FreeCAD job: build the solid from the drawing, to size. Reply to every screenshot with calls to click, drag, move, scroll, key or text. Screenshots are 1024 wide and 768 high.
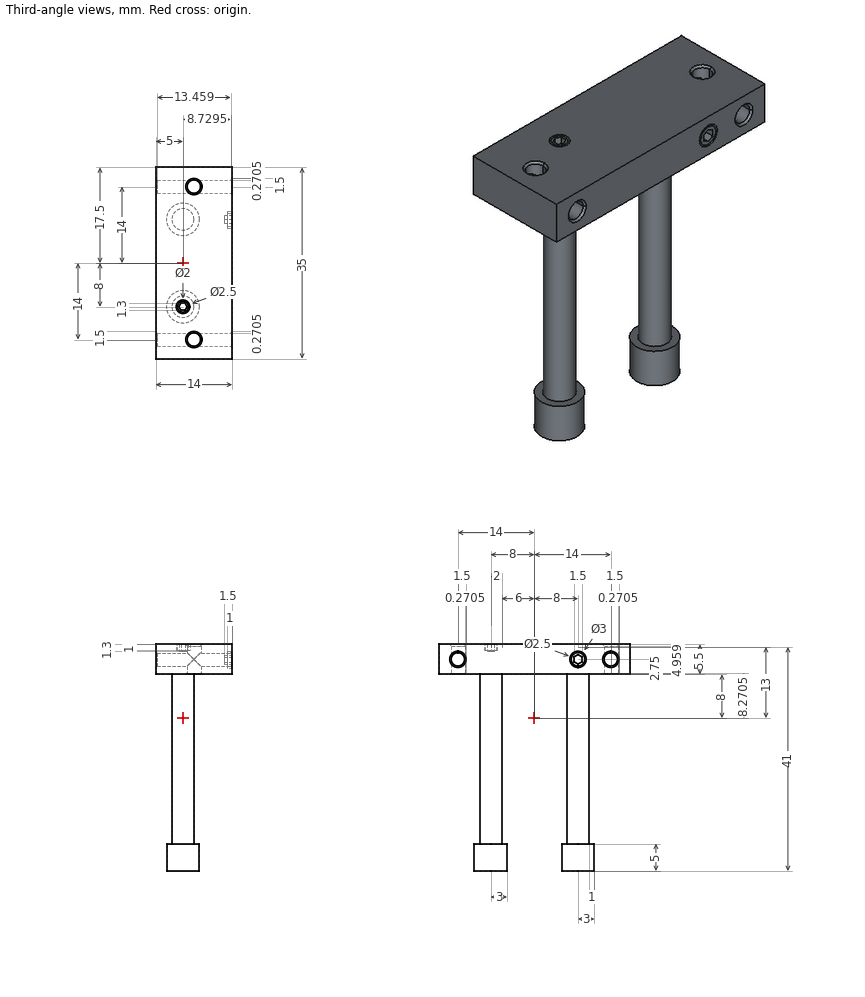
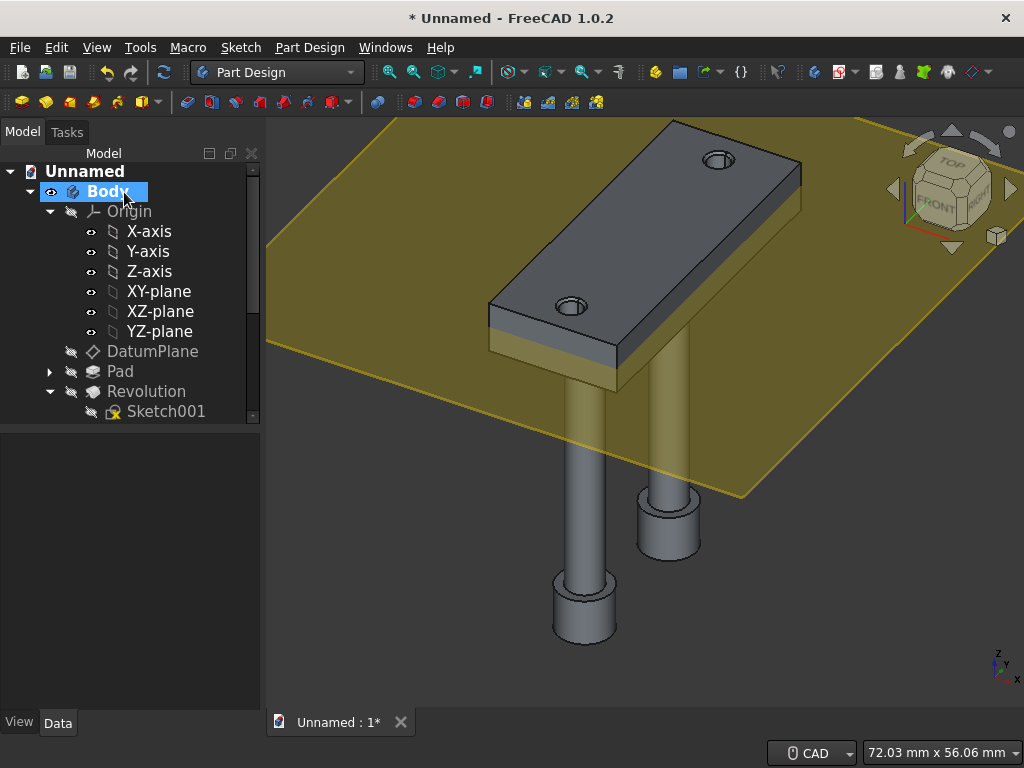
scroll(100, 287, down, 3)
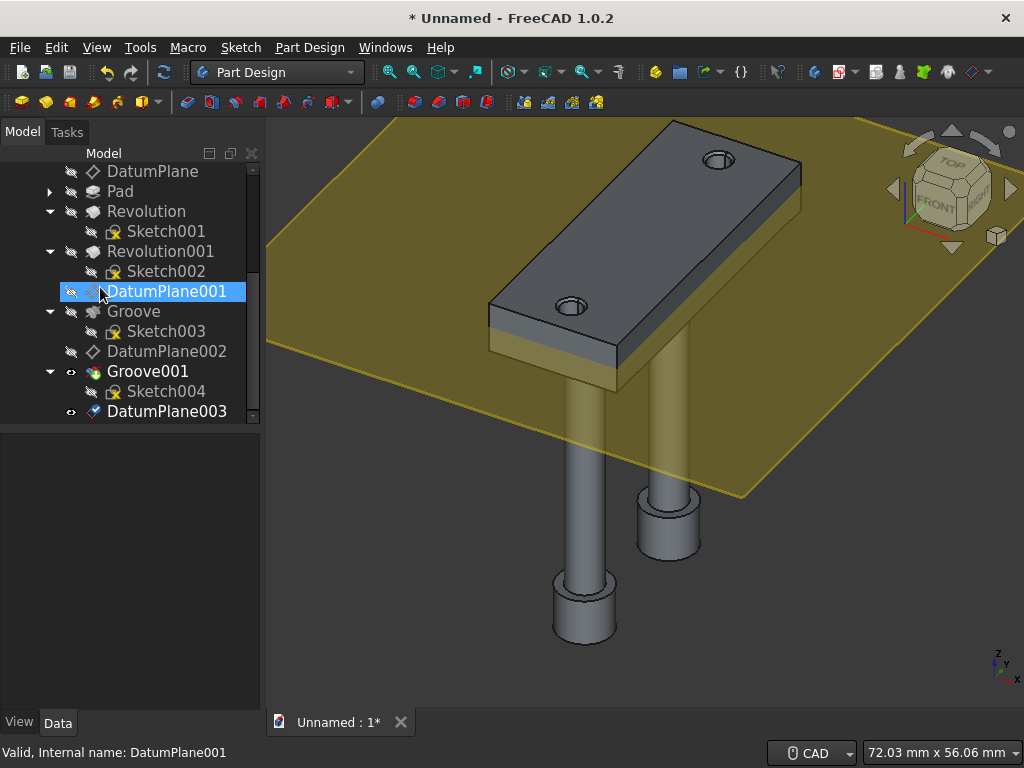
click(116, 412)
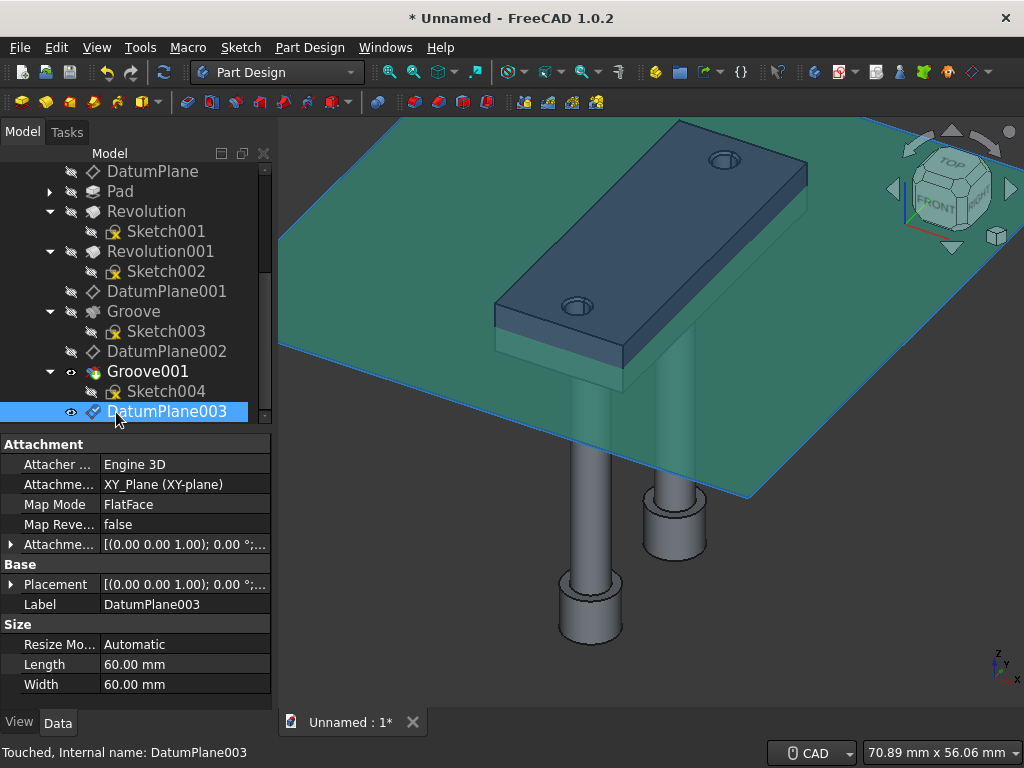
click(840, 72)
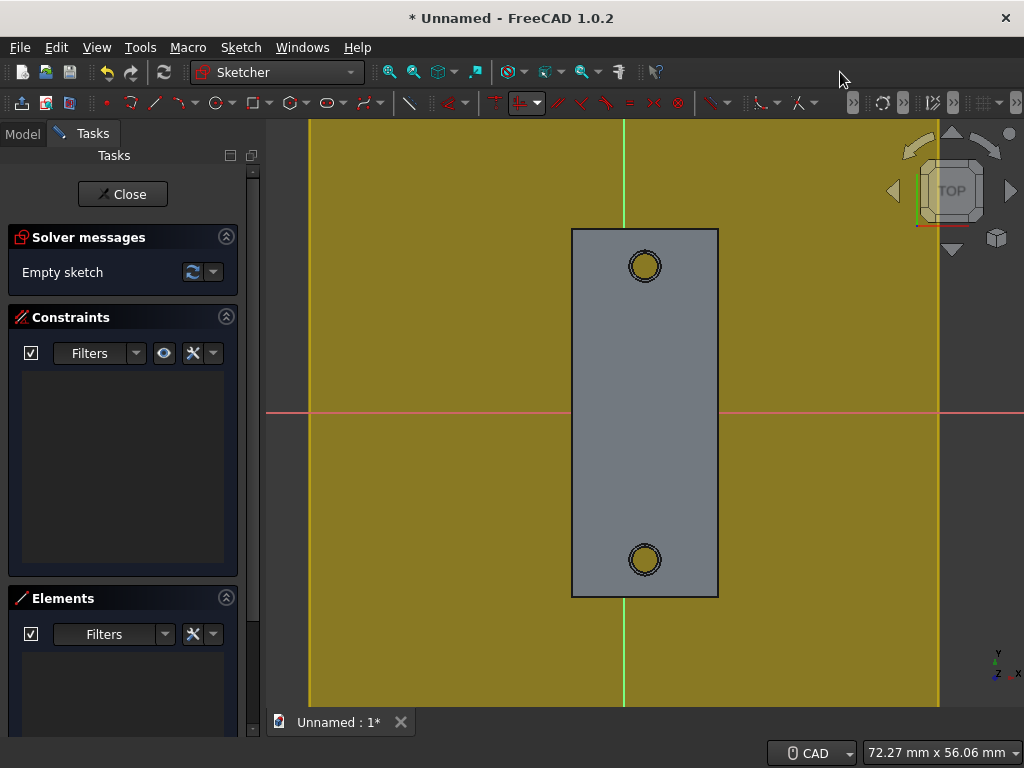
click(70, 104)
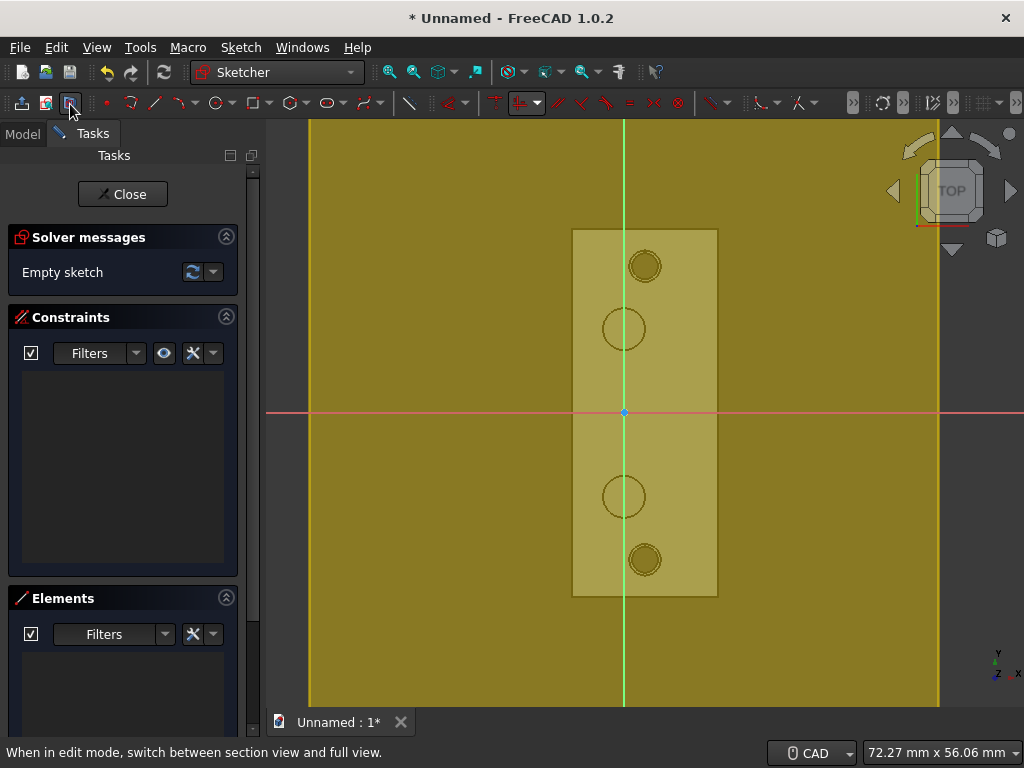
scroll(663, 233, up, 3)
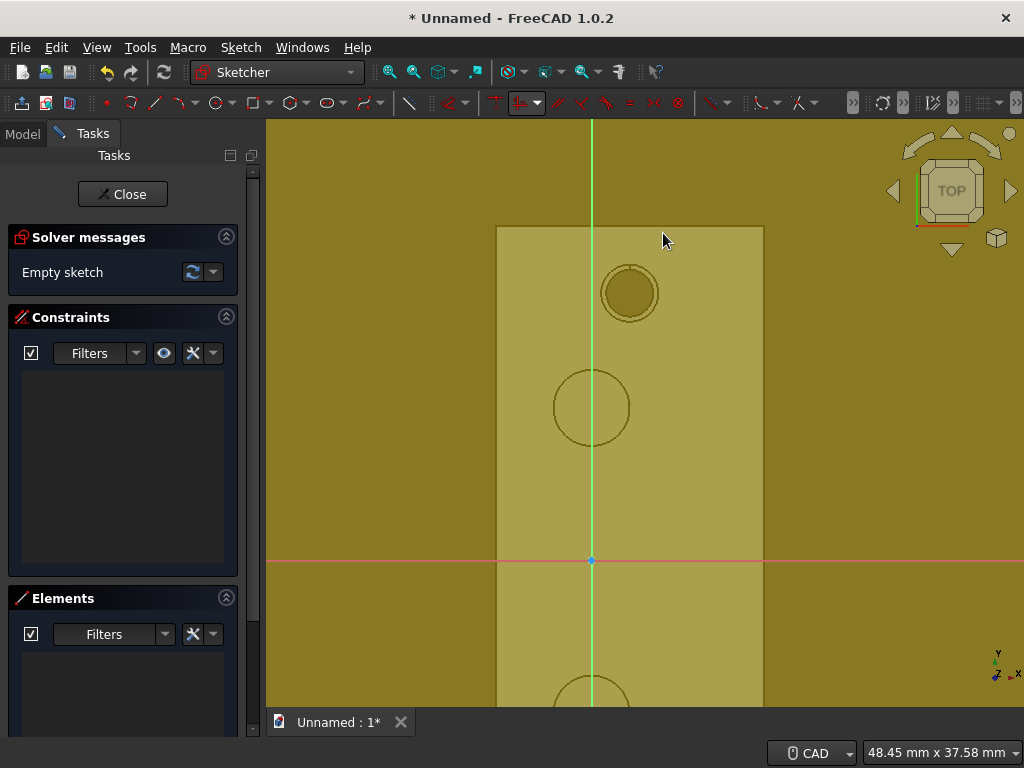
click(132, 104)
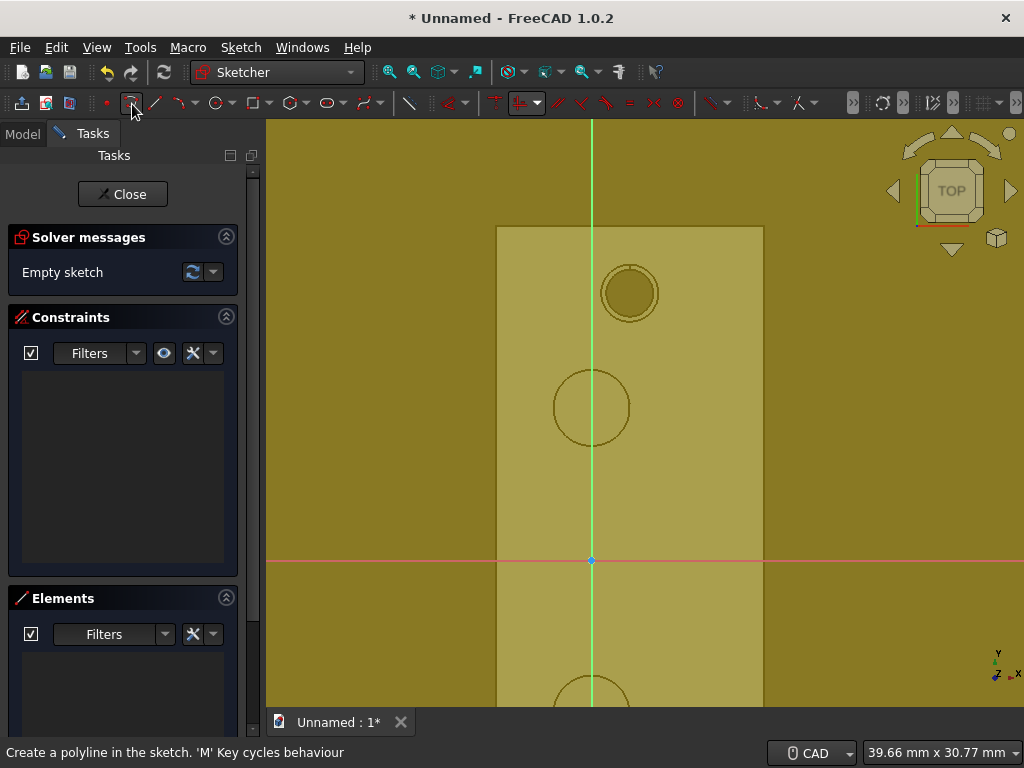
click(496, 293)
click(764, 293)
click(764, 265)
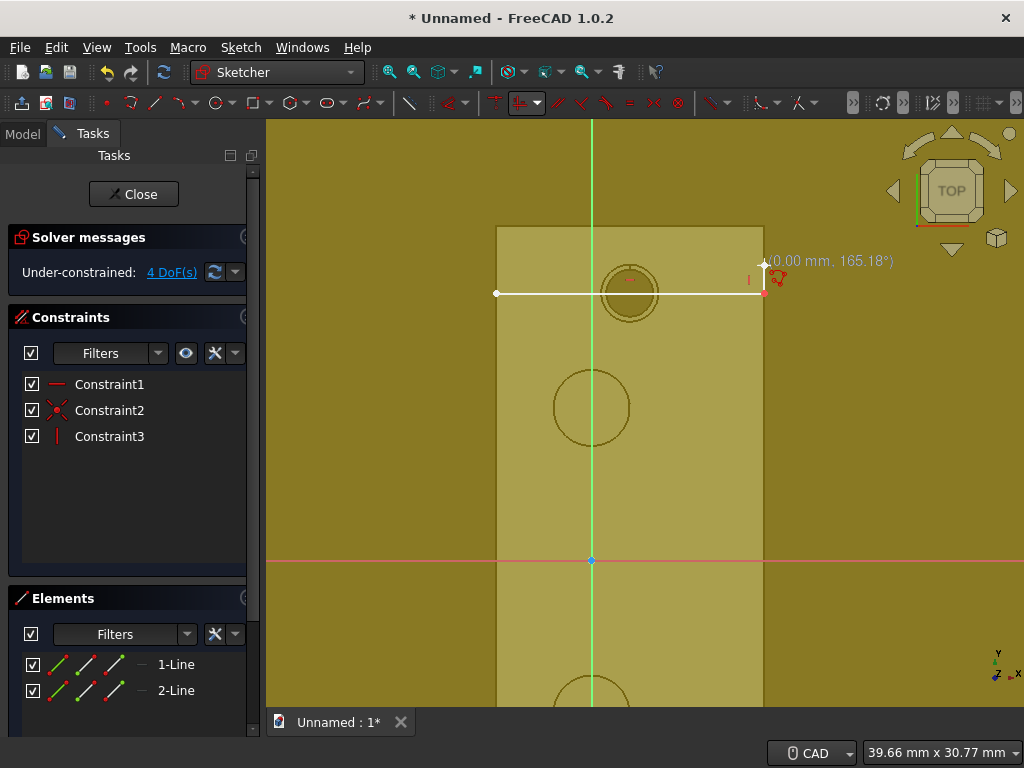
scroll(758, 270, up, 6)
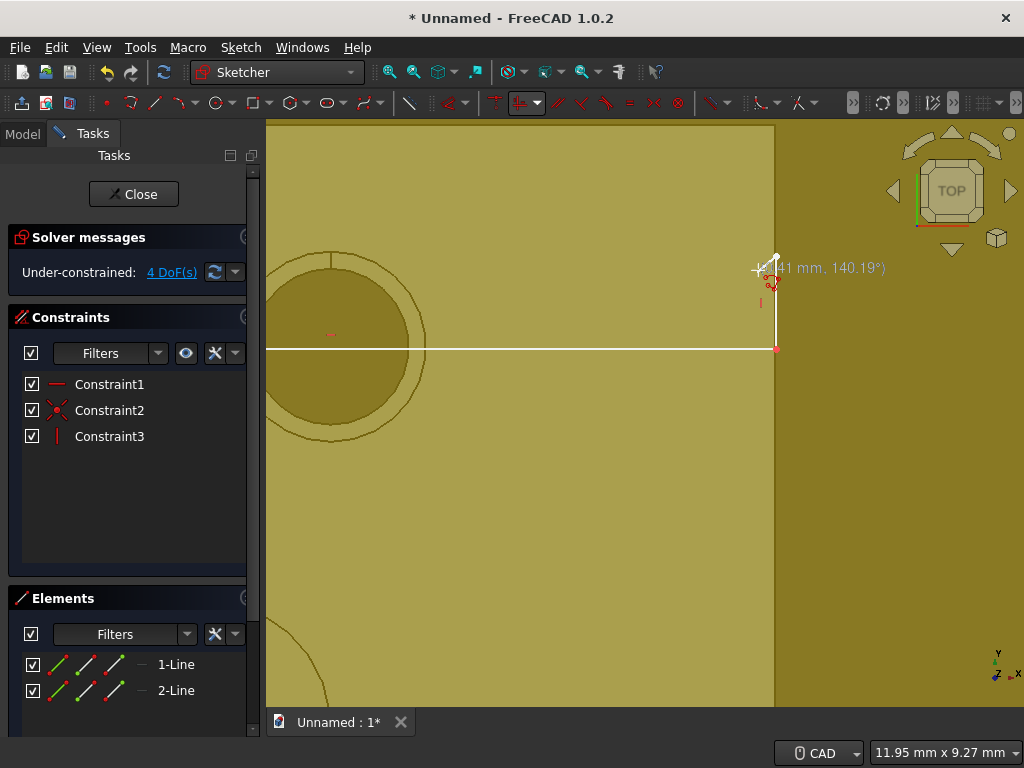
click(758, 269)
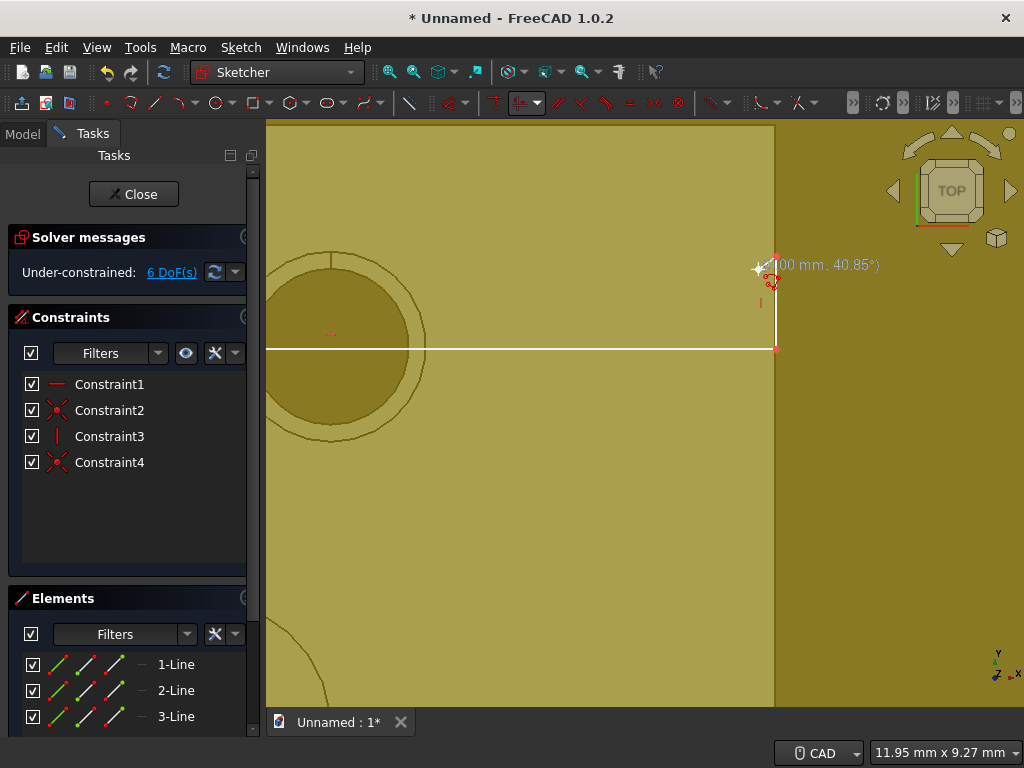
scroll(759, 271, down, 6)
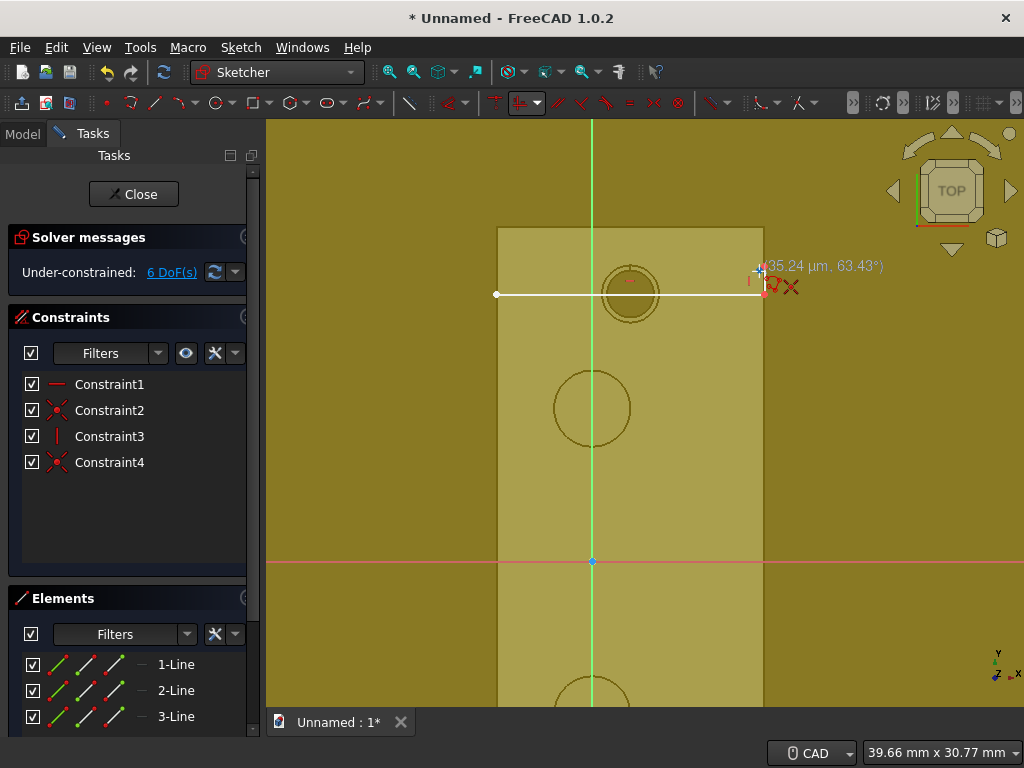
click(502, 271)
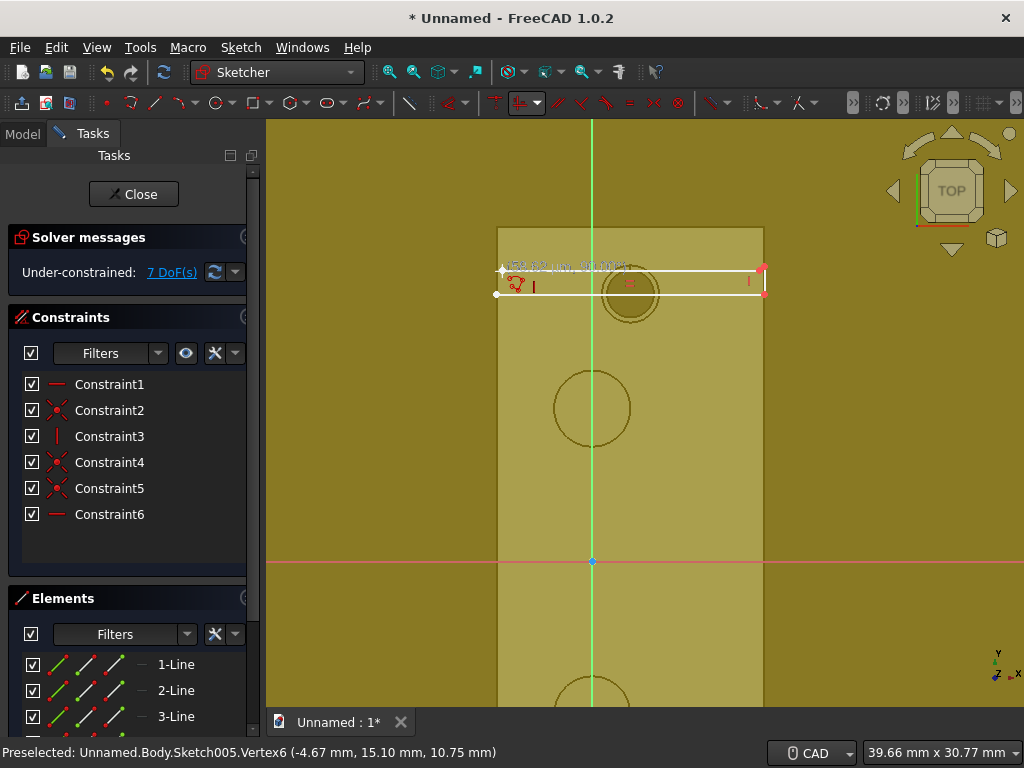
scroll(497, 265, up, 4)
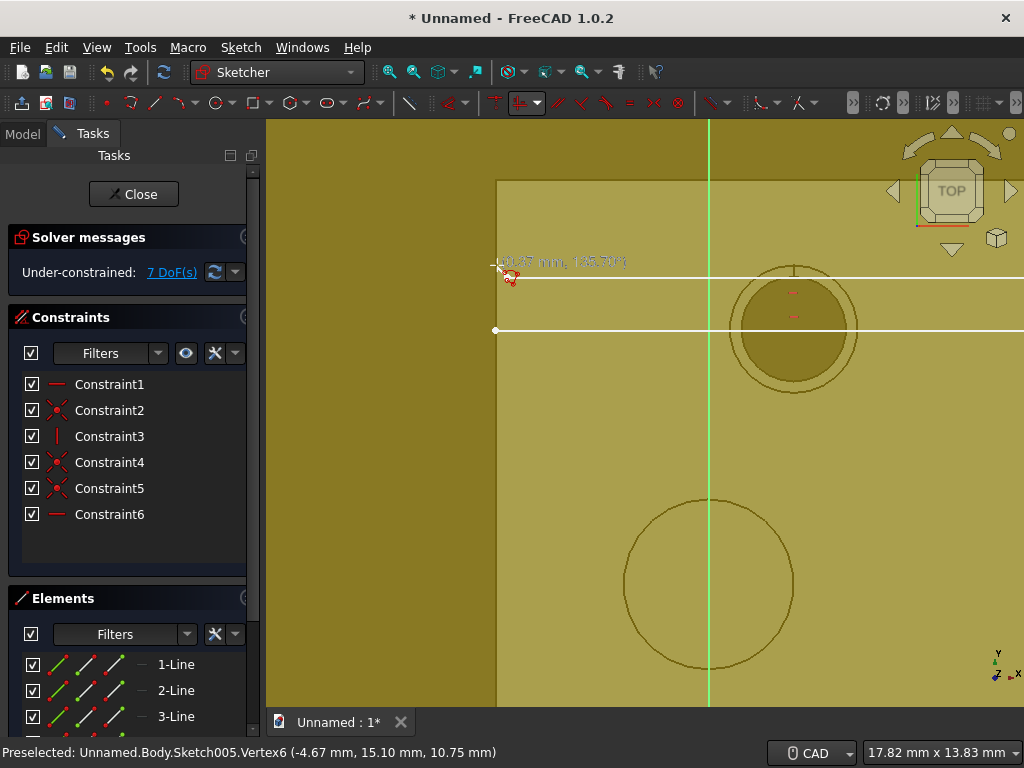
click(496, 265)
click(496, 331)